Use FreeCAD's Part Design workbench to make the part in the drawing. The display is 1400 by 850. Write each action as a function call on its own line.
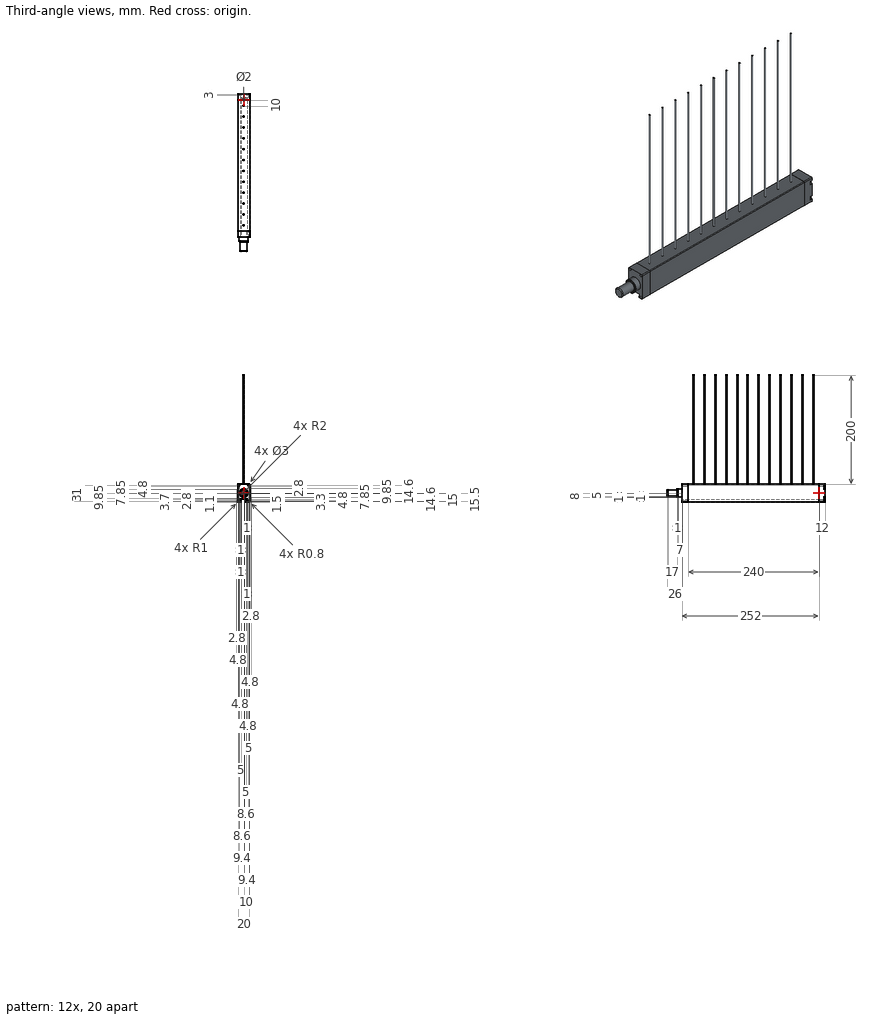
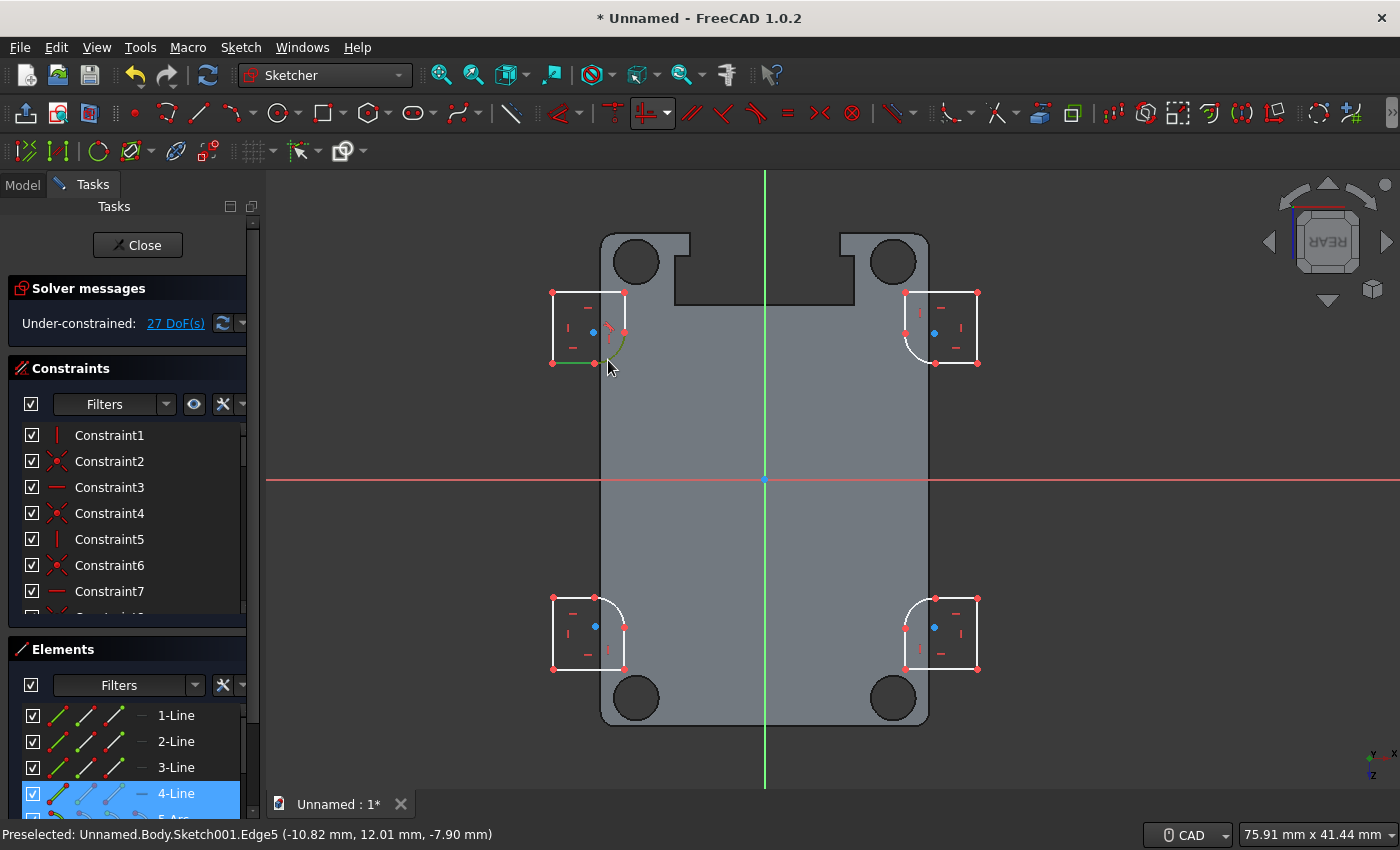
click(756, 114)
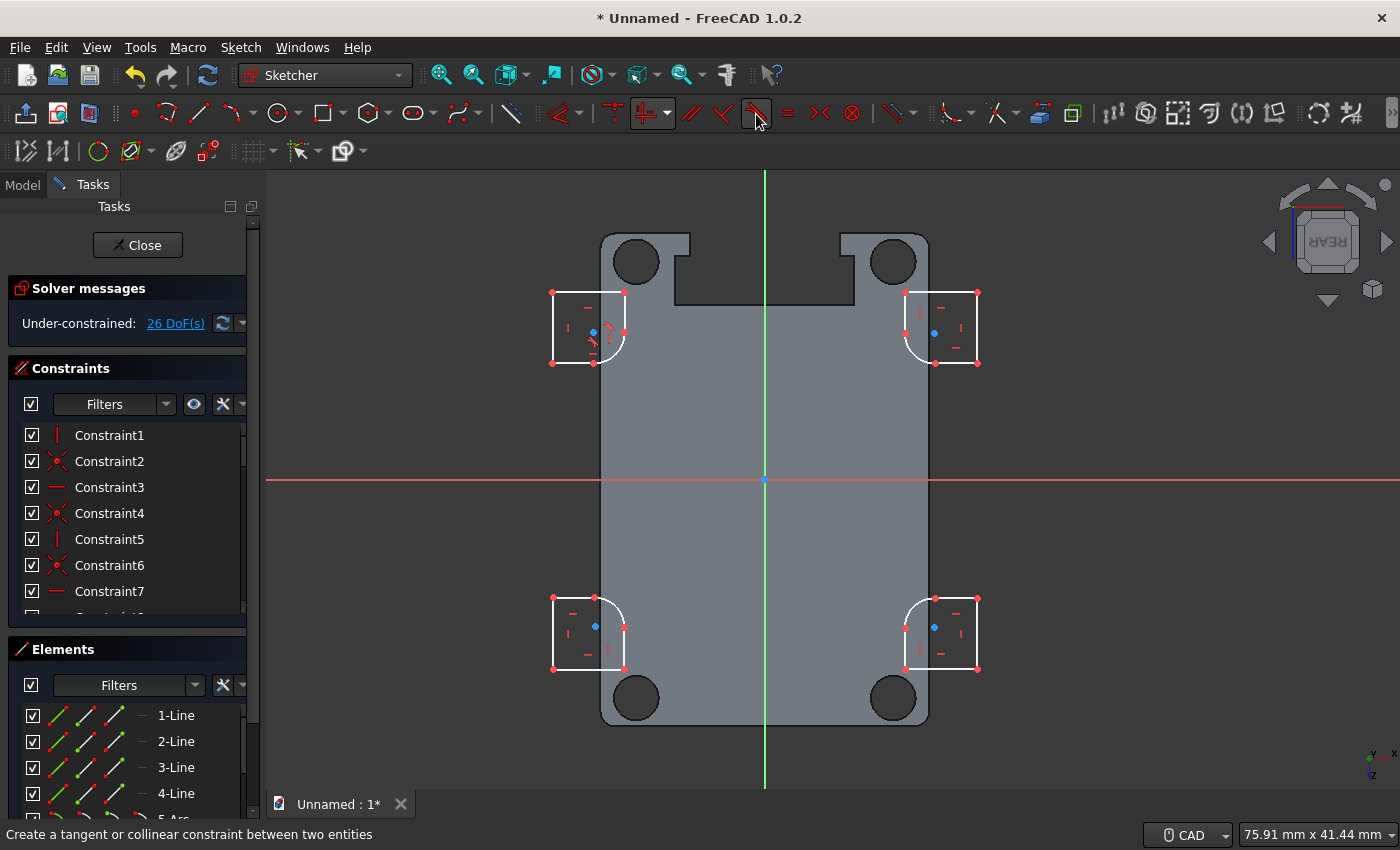
click(948, 363)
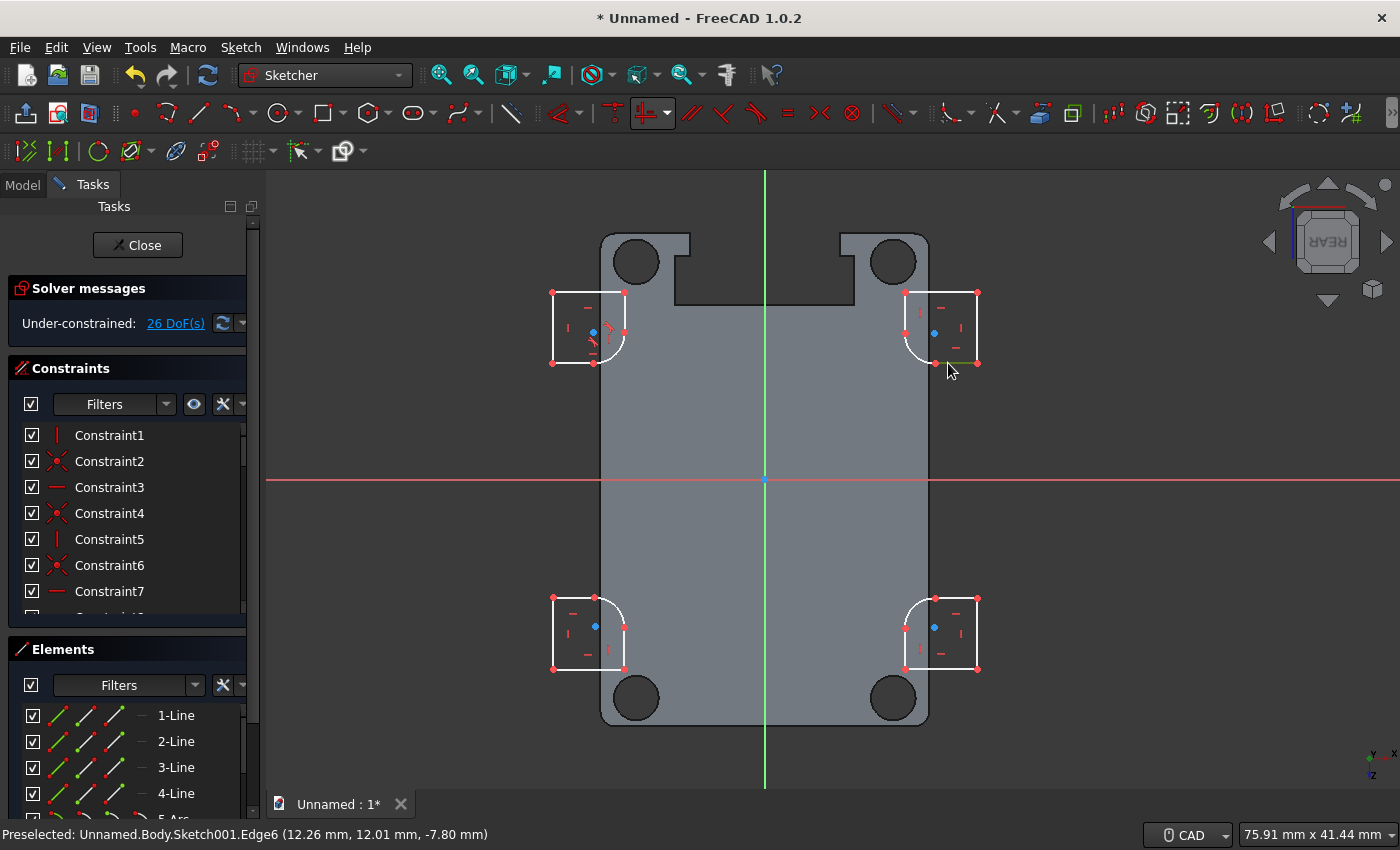
click(908, 347)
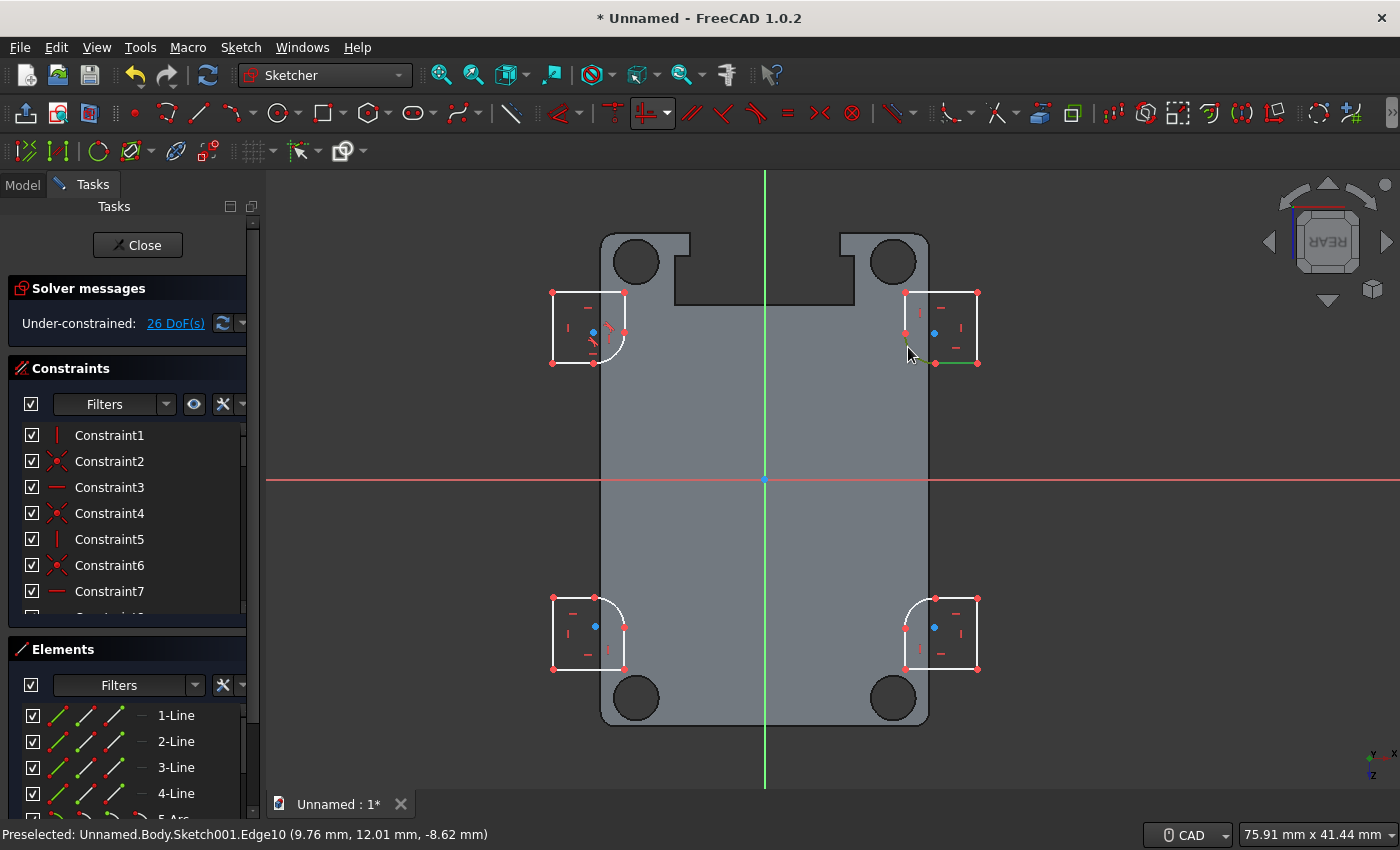
click(756, 114)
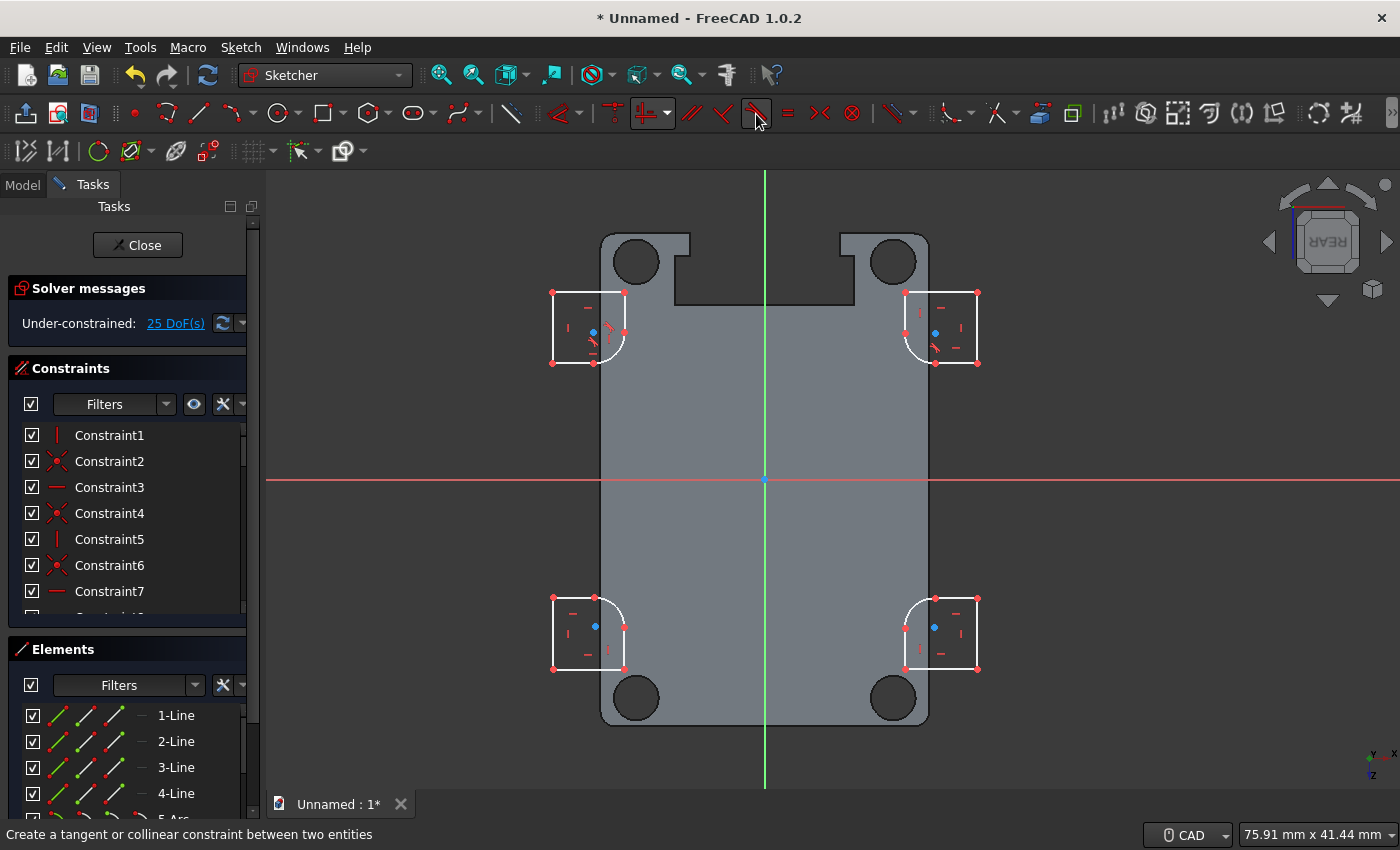
click(905, 305)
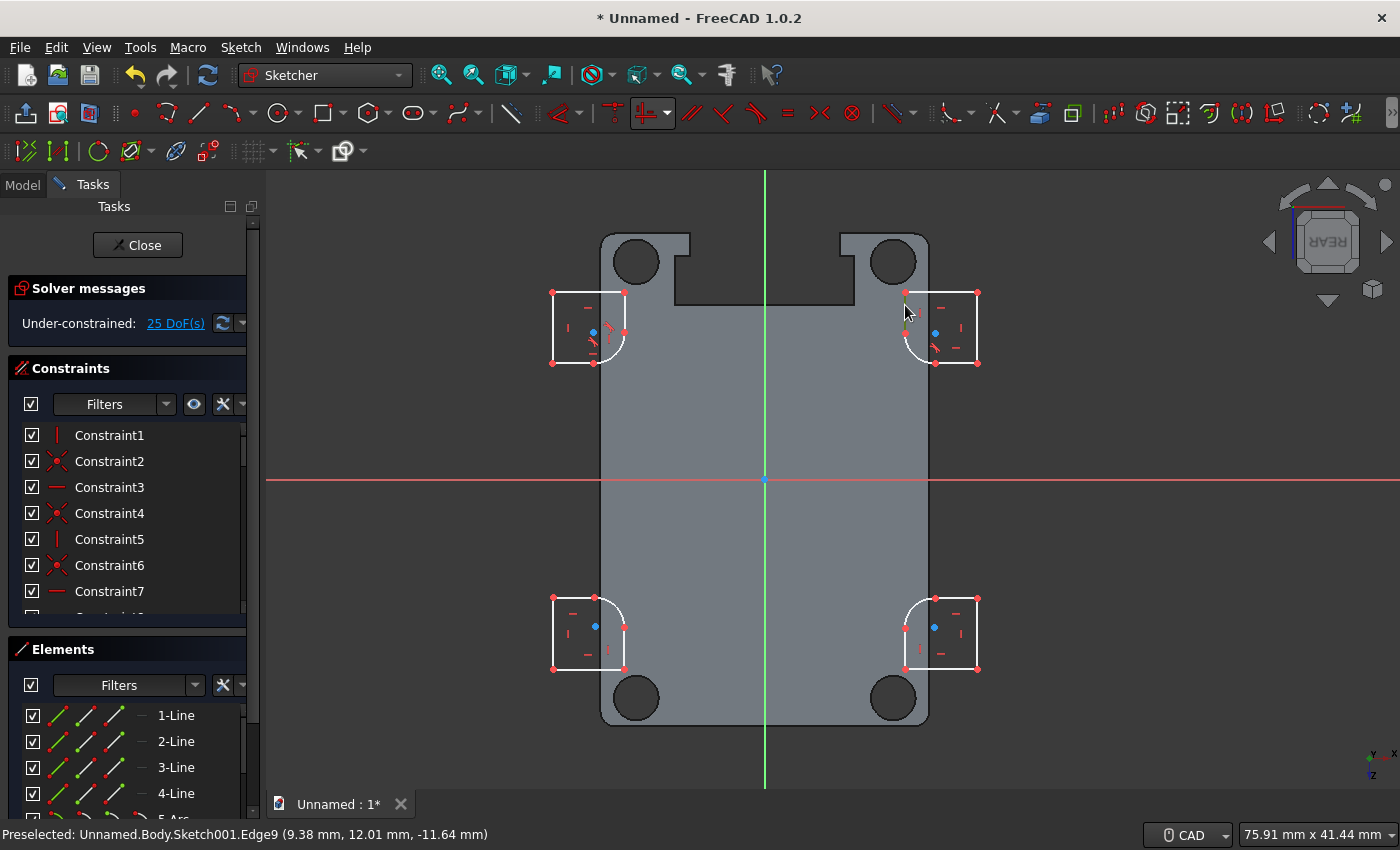
click(908, 347)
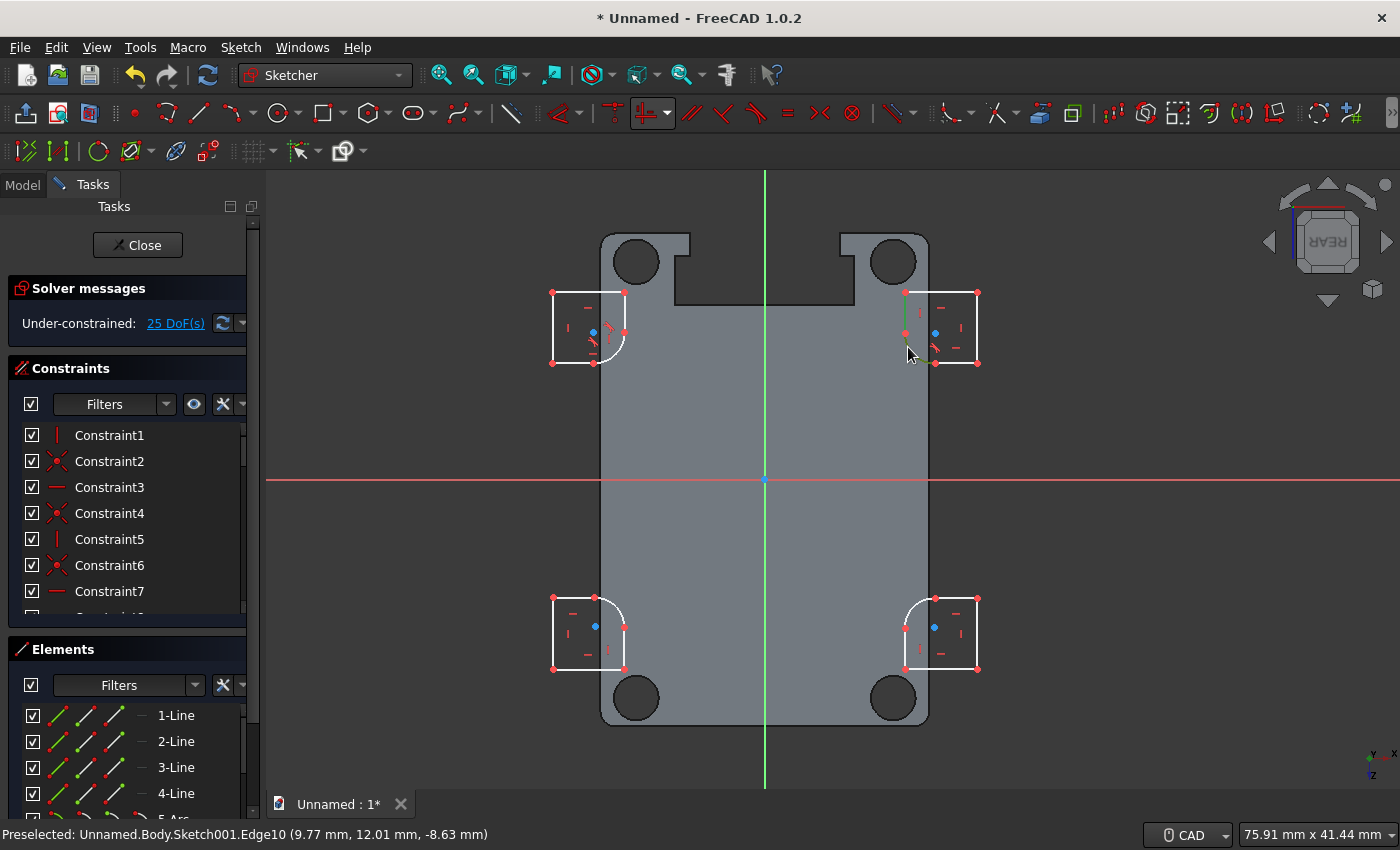
key(t)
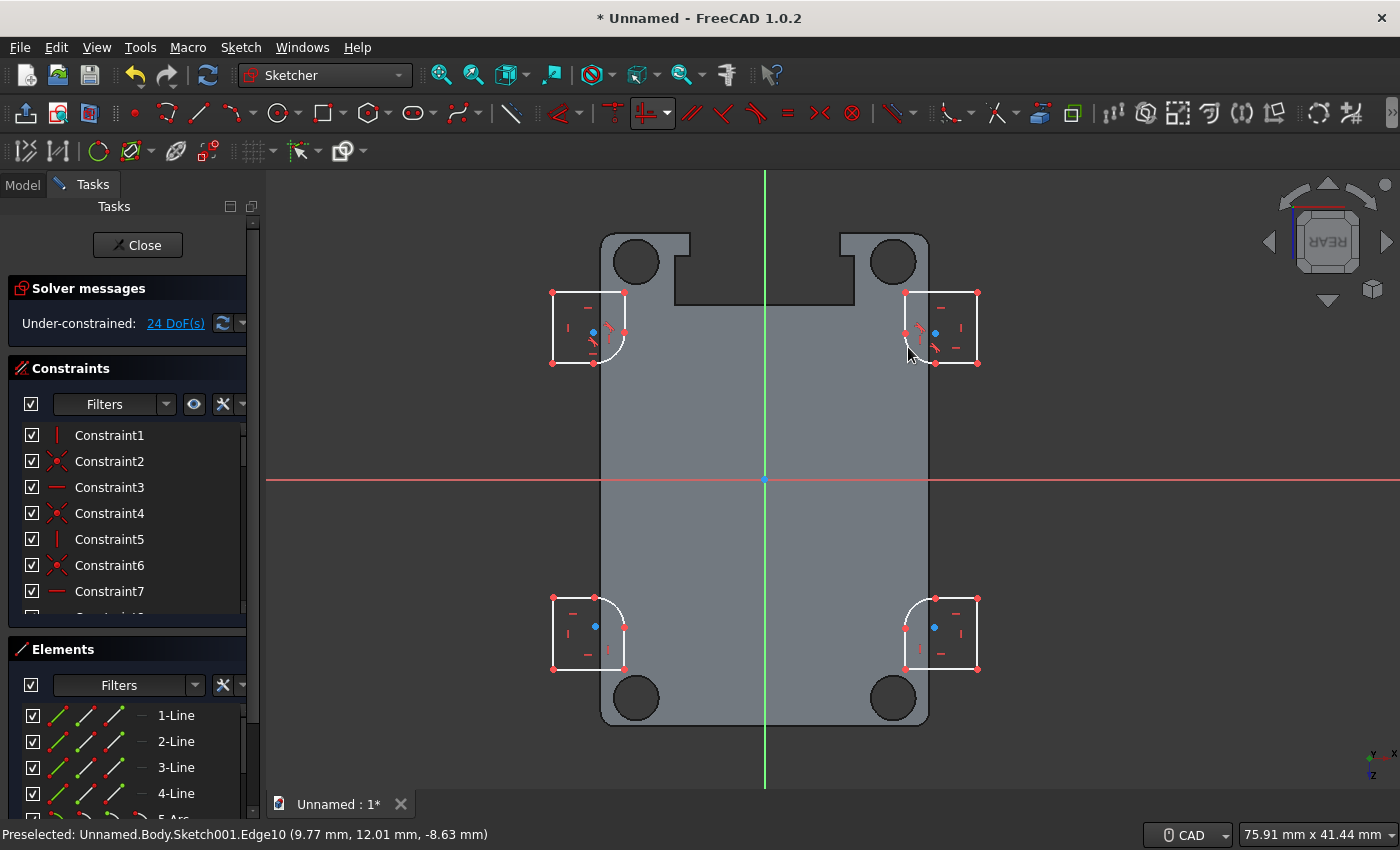
click(905, 641)